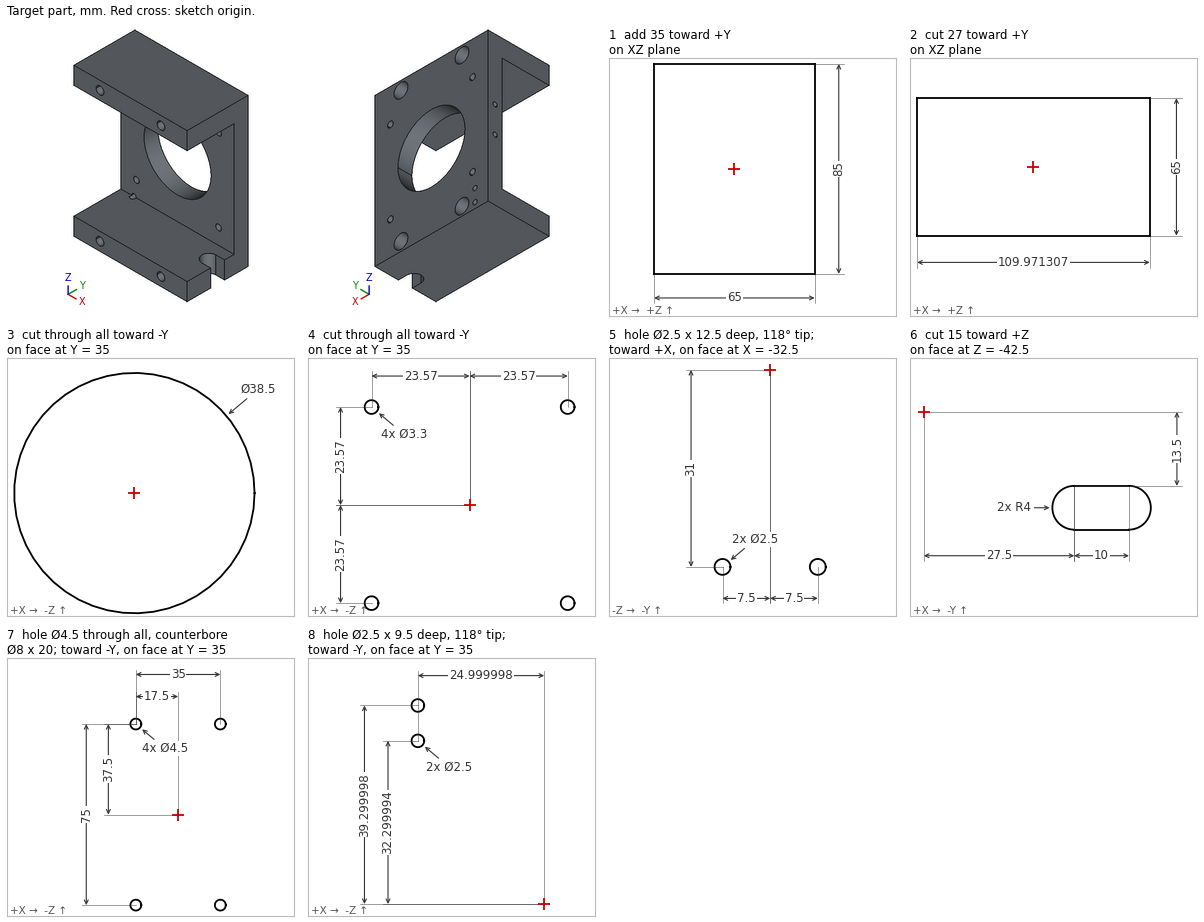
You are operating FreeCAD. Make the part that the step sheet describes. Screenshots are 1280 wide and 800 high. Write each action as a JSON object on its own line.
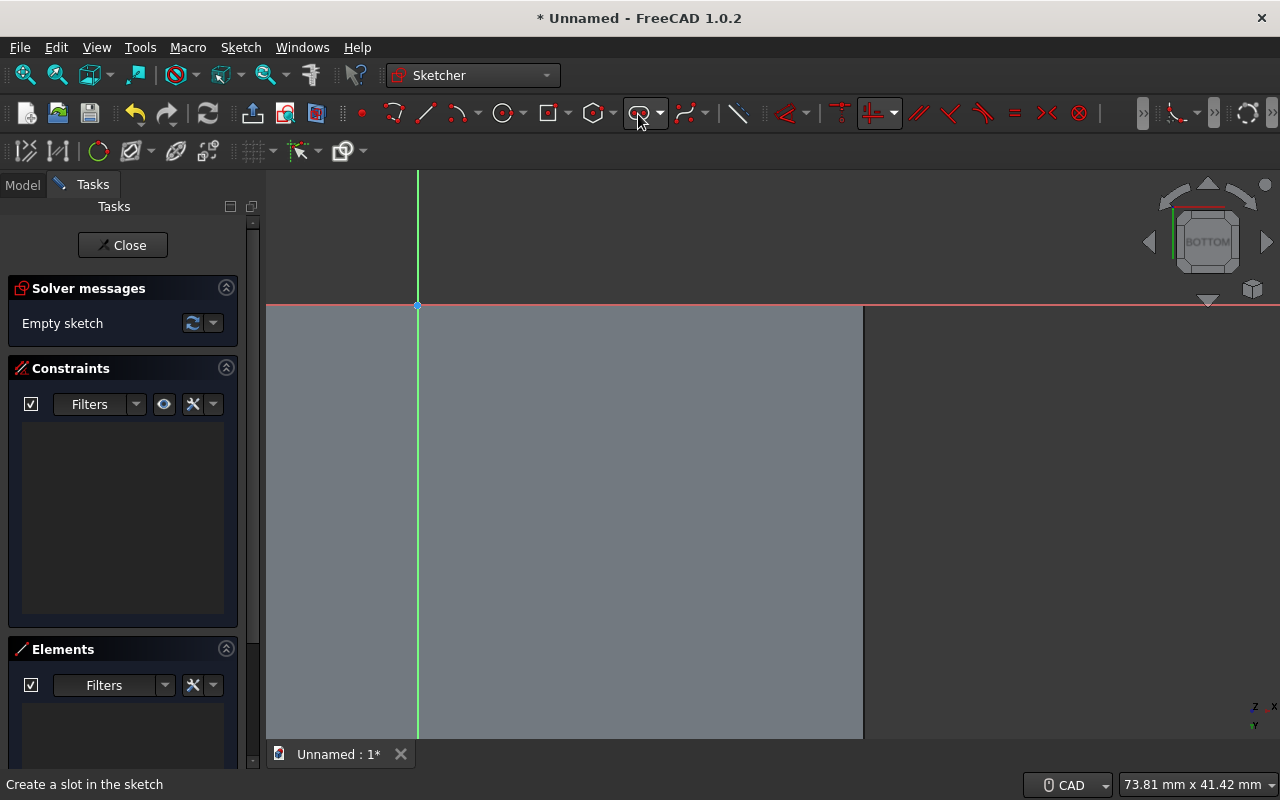
{"action": "left_click", "coordinate": [796, 546]}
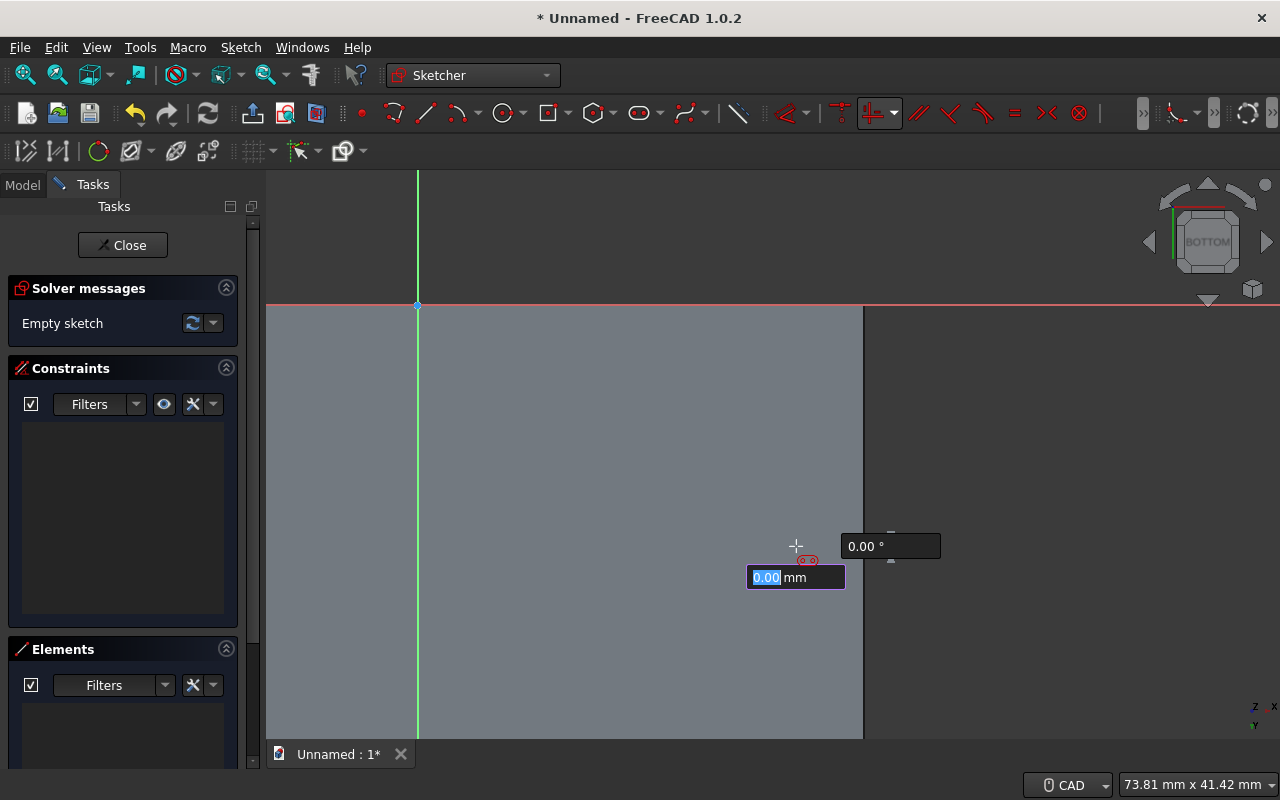
{"action": "left_click", "coordinate": [933, 546]}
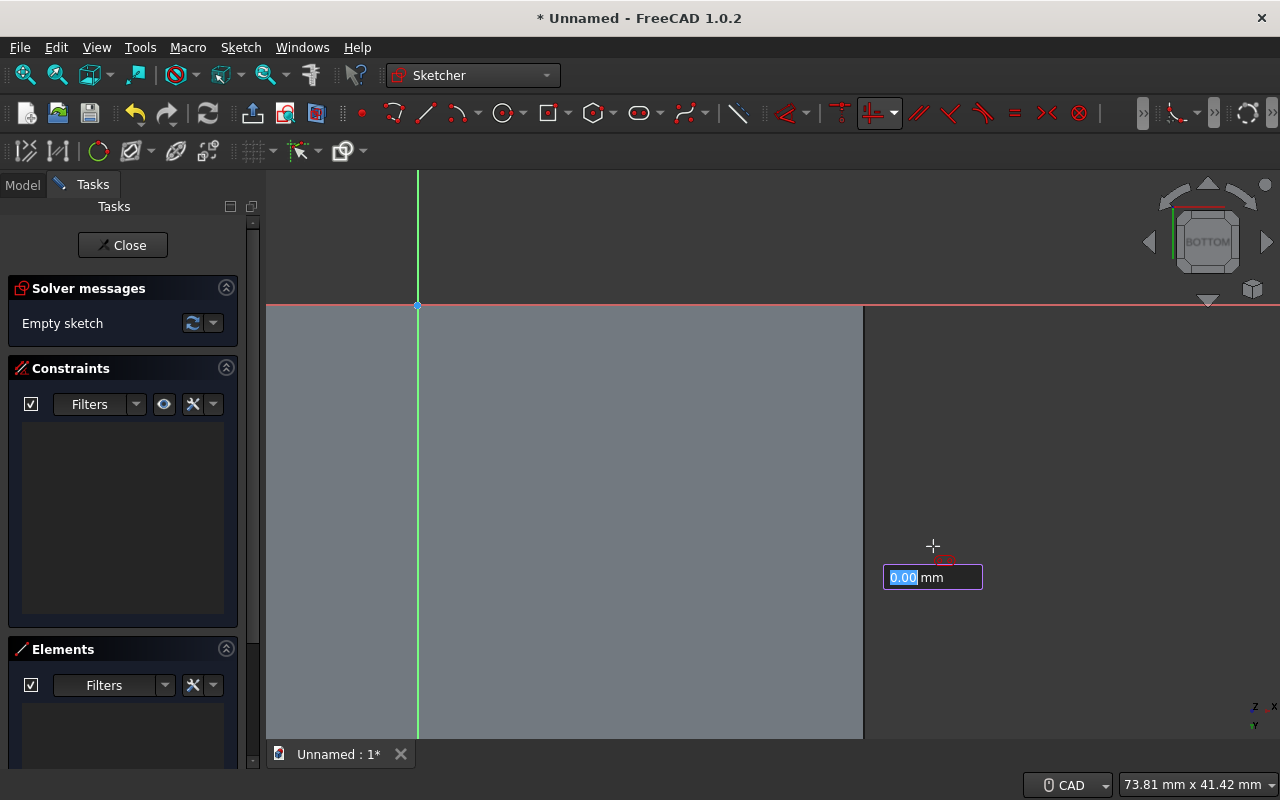
{"action": "left_click", "coordinate": [864, 491]}
{"action": "key", "text": "Escape"}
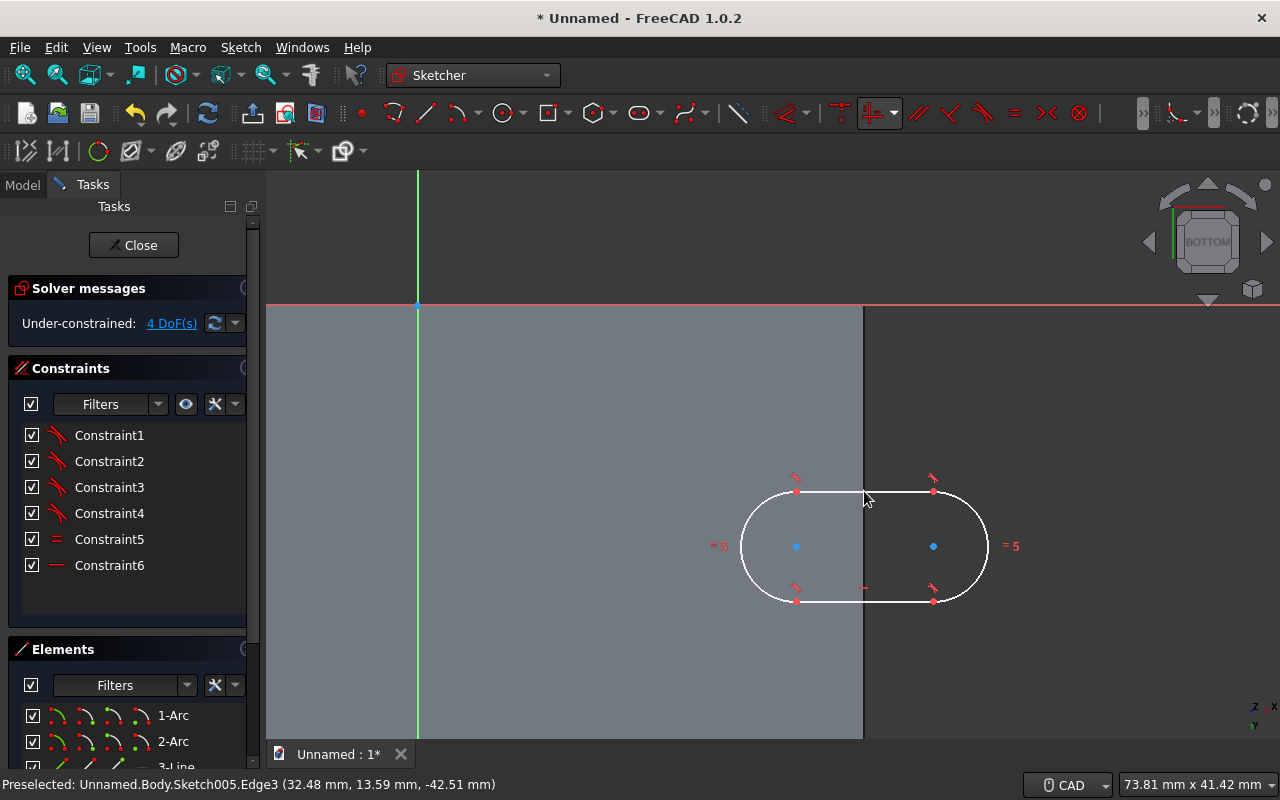
{"action": "left_click", "coordinate": [786, 114]}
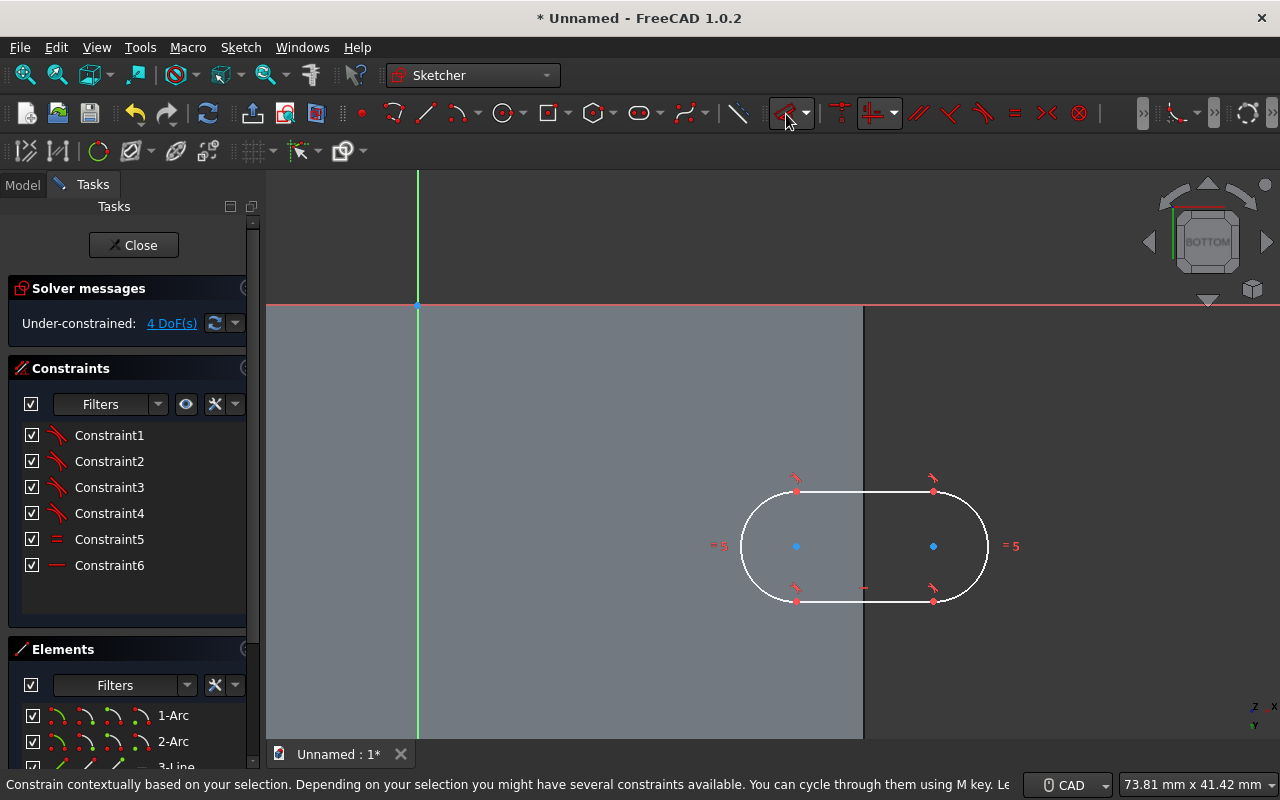
{"action": "left_click", "coordinate": [752, 515]}
{"action": "left_click", "coordinate": [726, 496]}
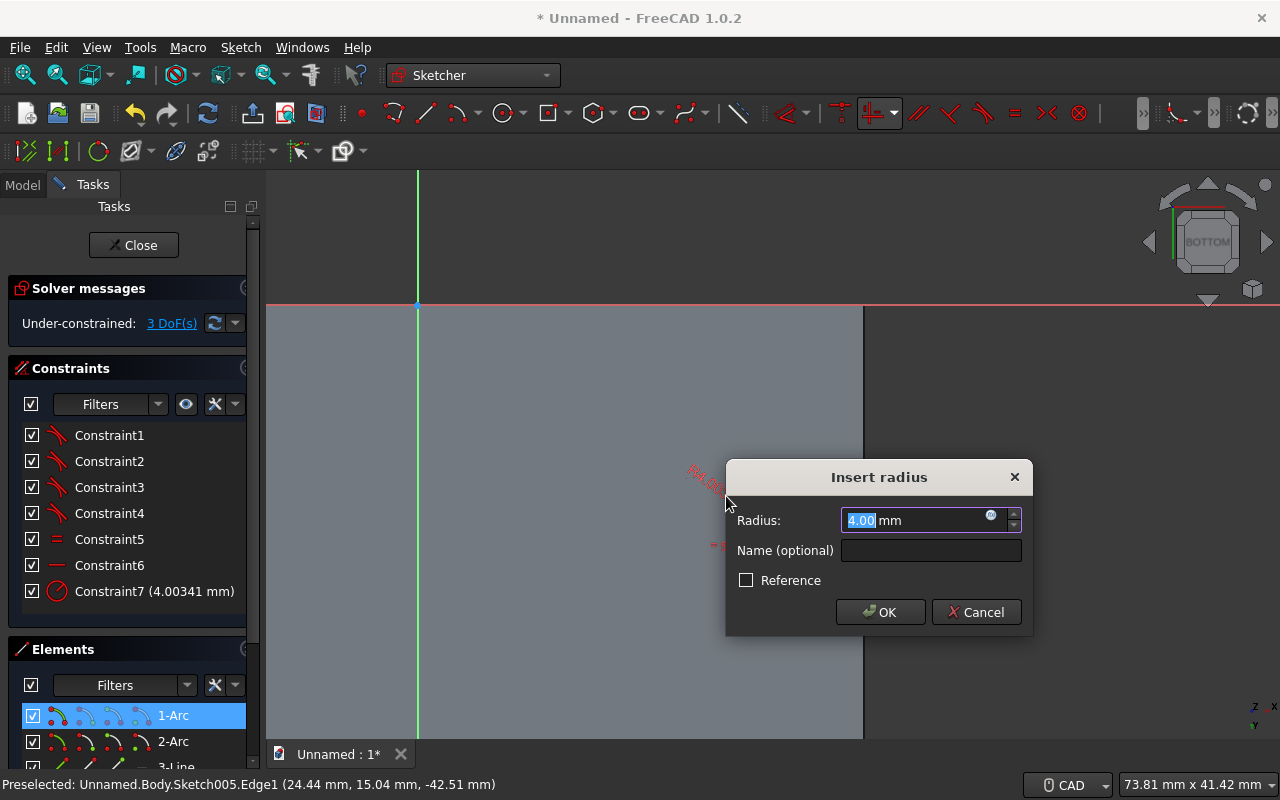
{"action": "type", "text": "4"}
{"action": "key", "text": "Return"}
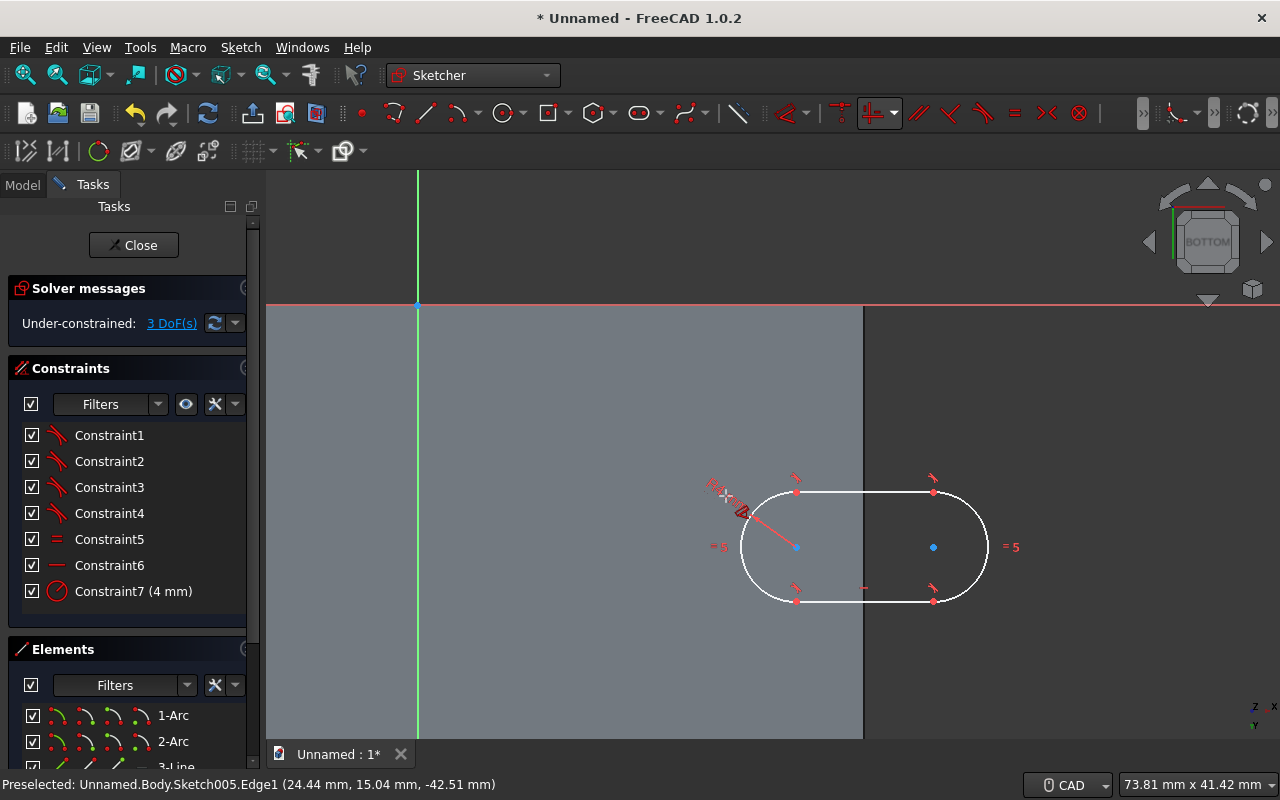
{"action": "left_click", "coordinate": [837, 492]}
{"action": "left_click", "coordinate": [864, 526]}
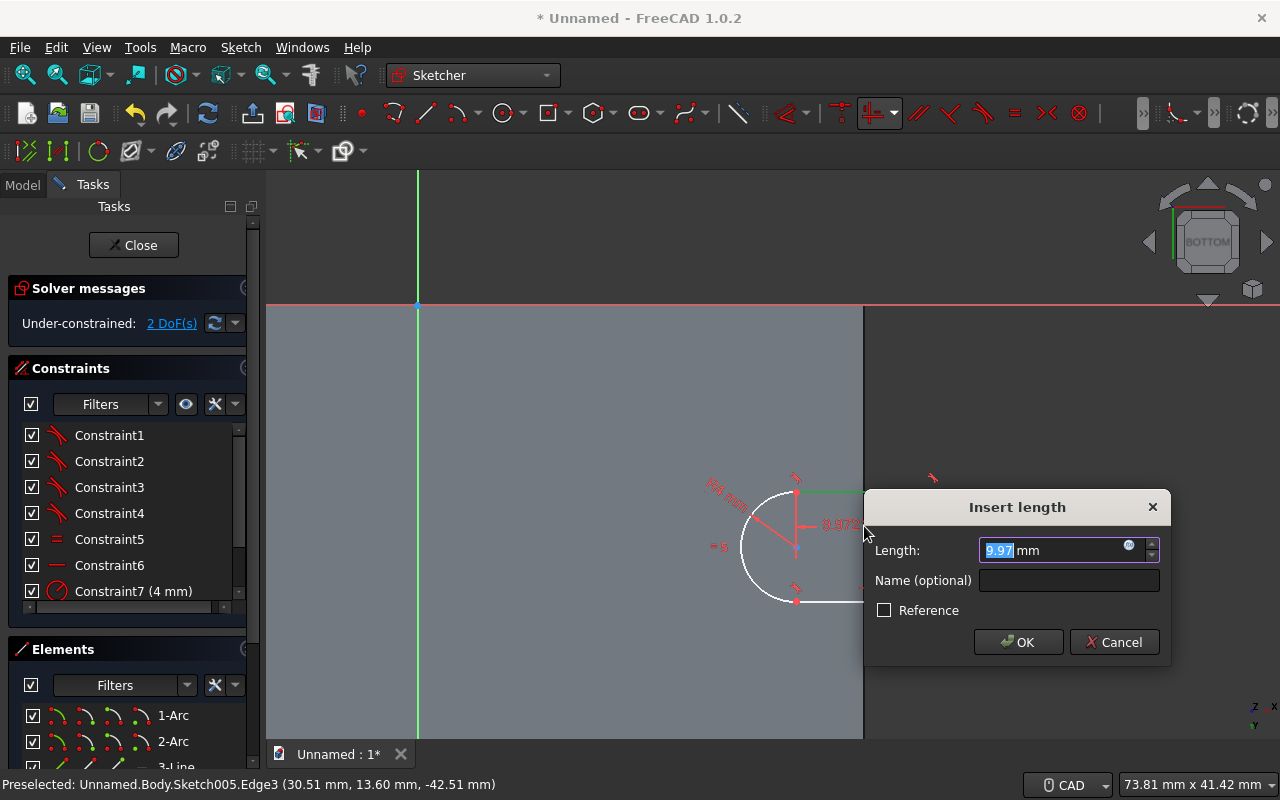
{"action": "type", "text": "10"}
{"action": "key", "text": "Return"}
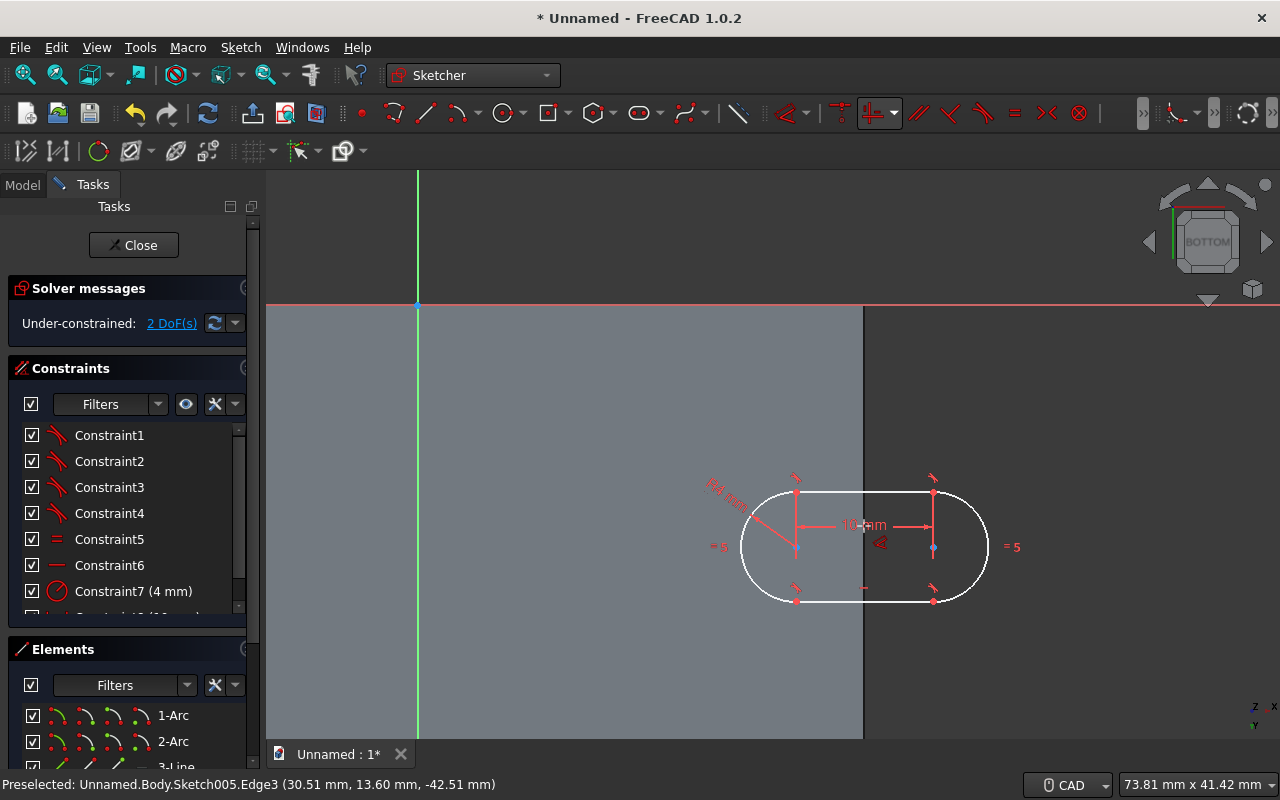
{"action": "left_click", "coordinate": [796, 492]}
{"action": "left_click", "coordinate": [607, 271]}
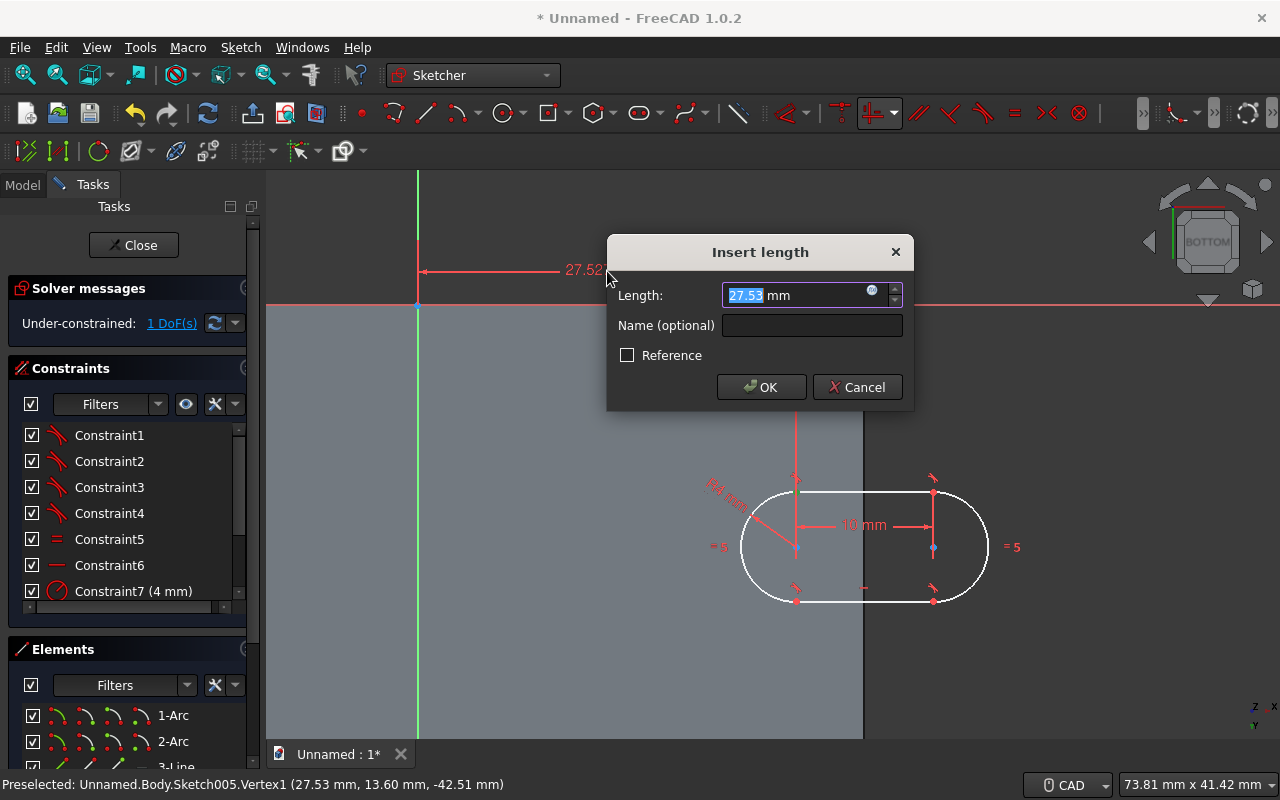
{"action": "type", "text": "27.5"}
{"action": "key", "text": "Return"}